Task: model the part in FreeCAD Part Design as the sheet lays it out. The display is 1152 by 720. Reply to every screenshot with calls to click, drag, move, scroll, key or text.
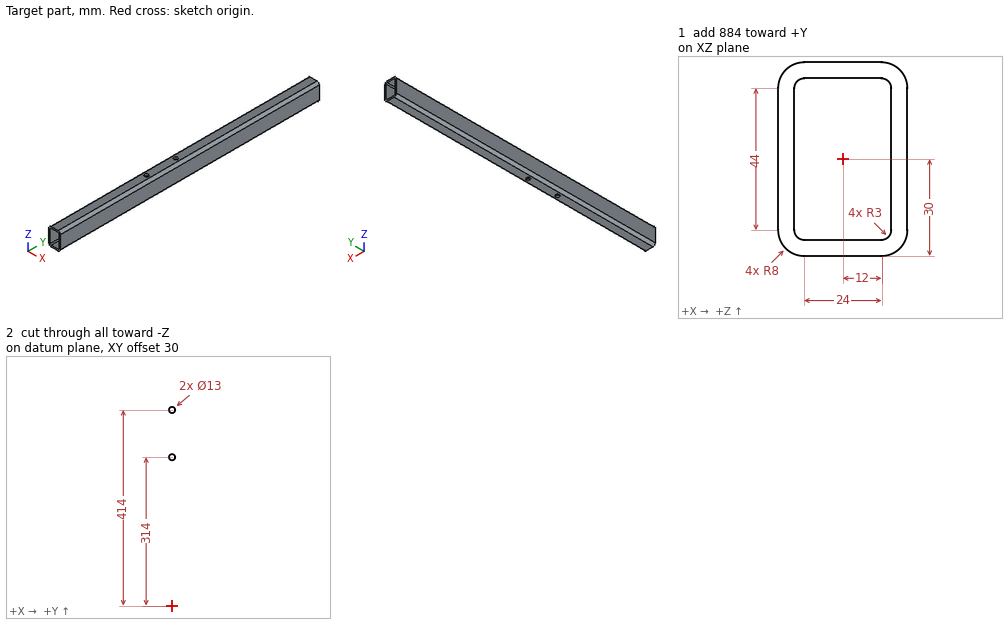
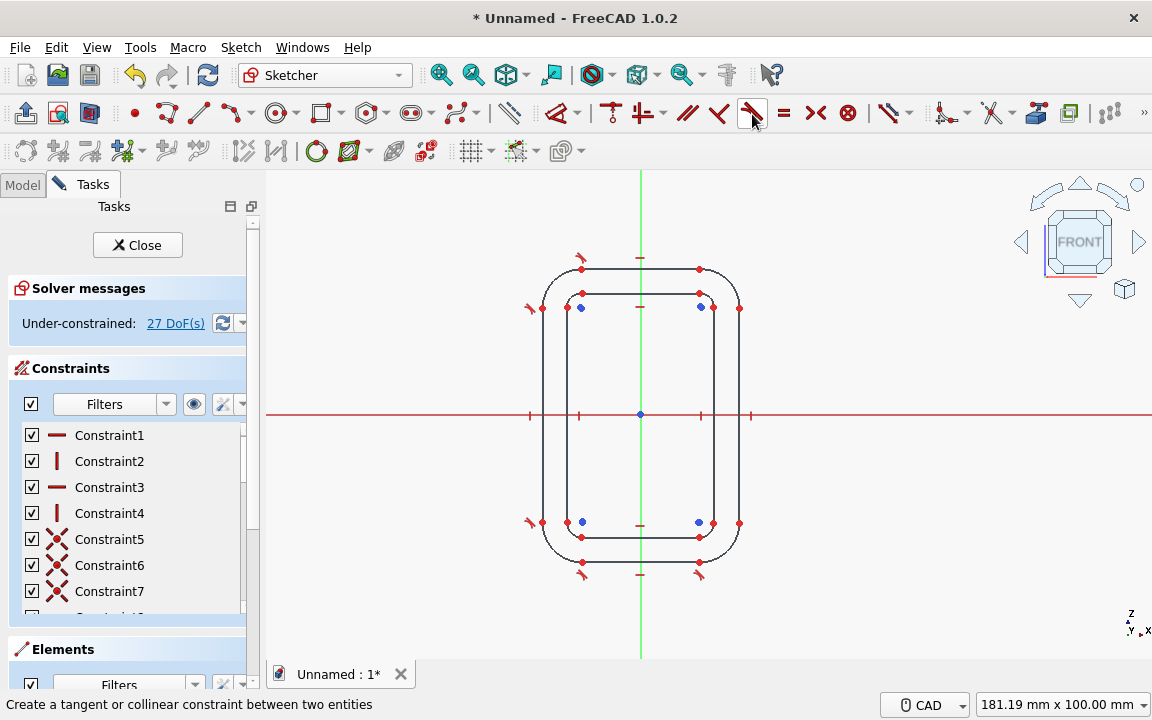
click(617, 269)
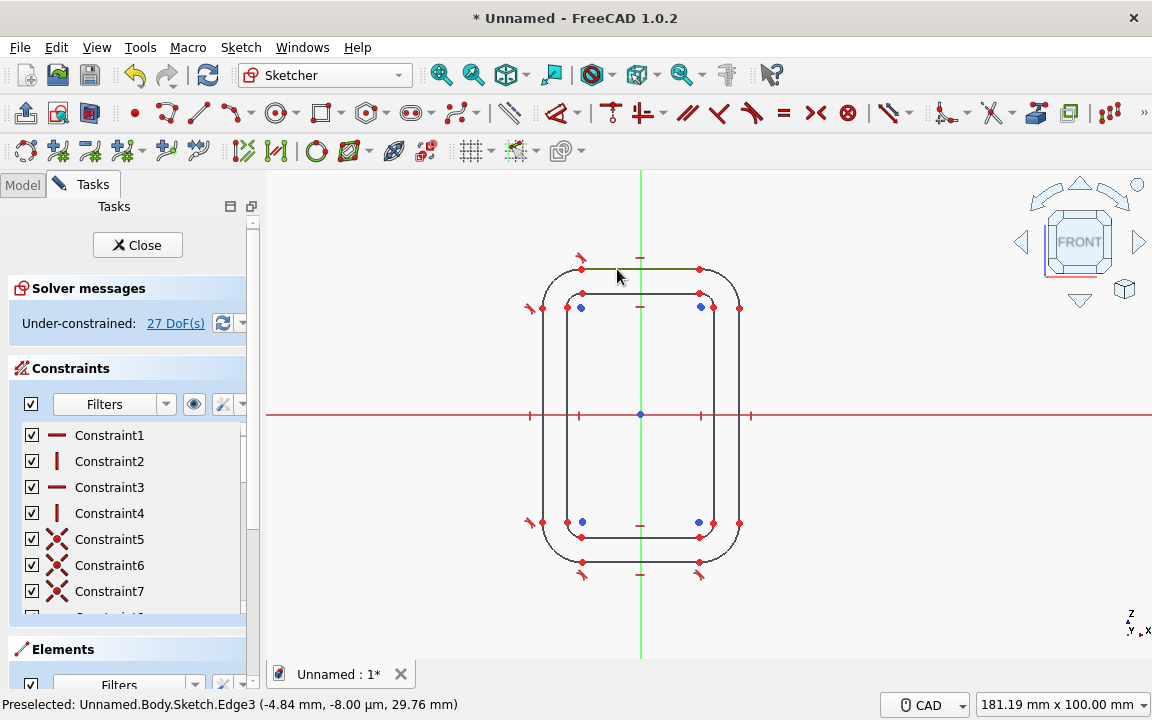
click(735, 290)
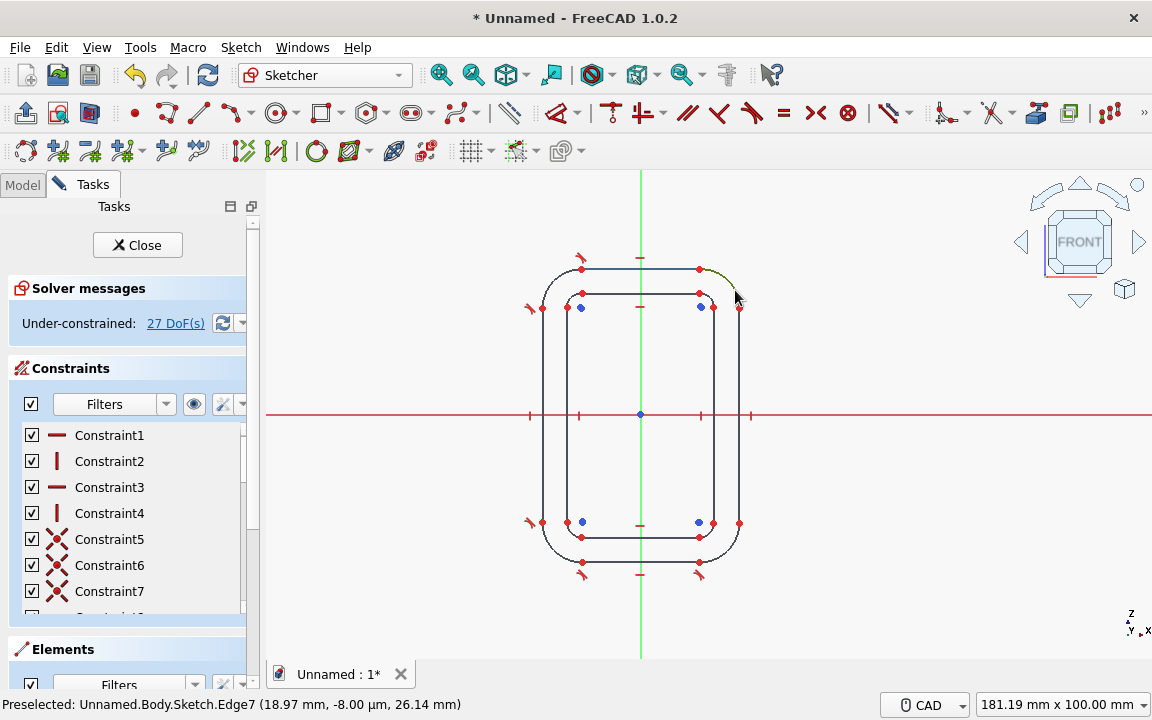
key(t)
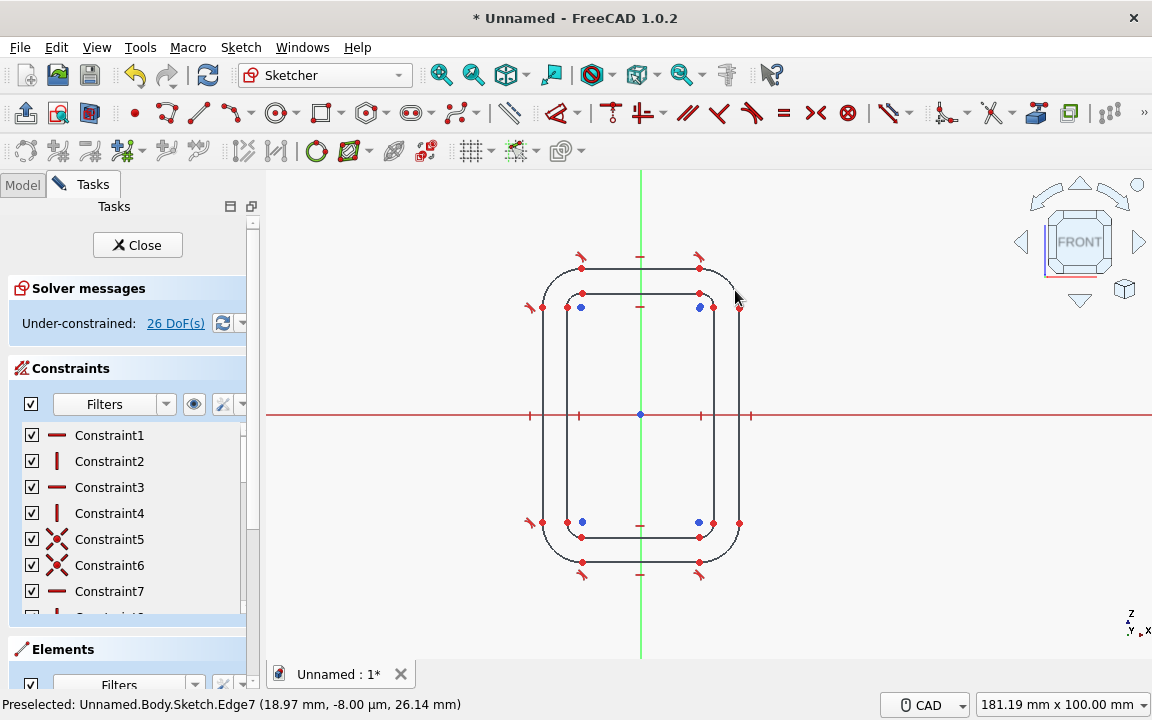
click(739, 373)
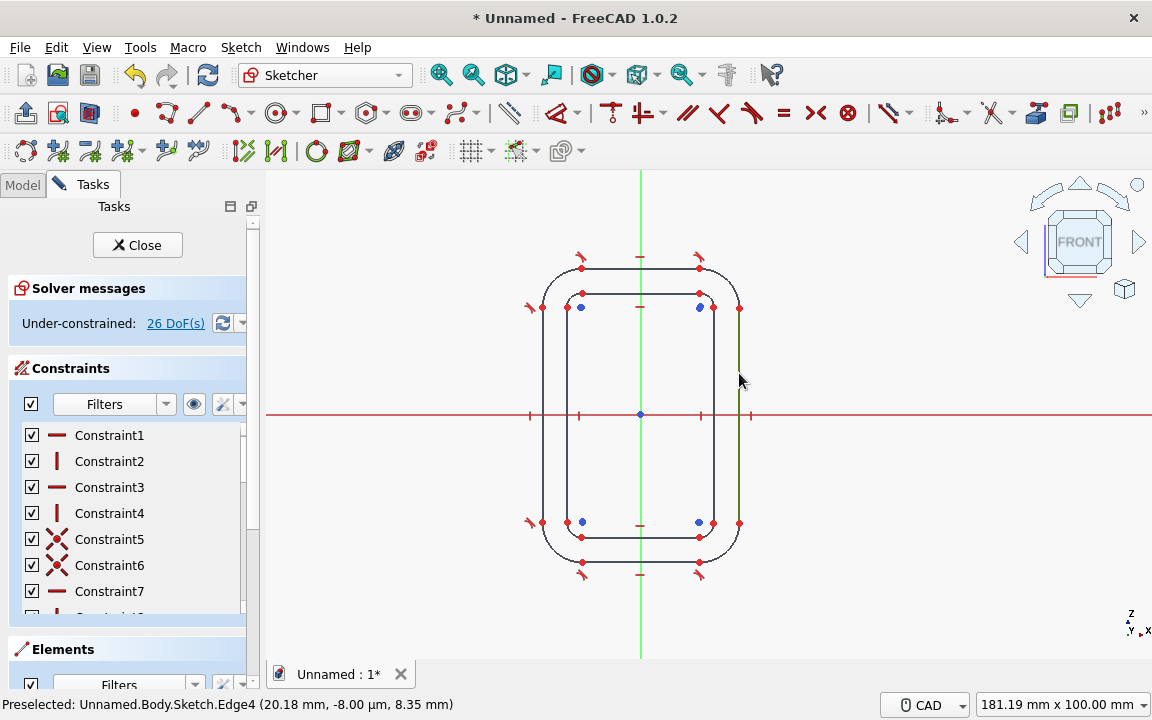
click(735, 290)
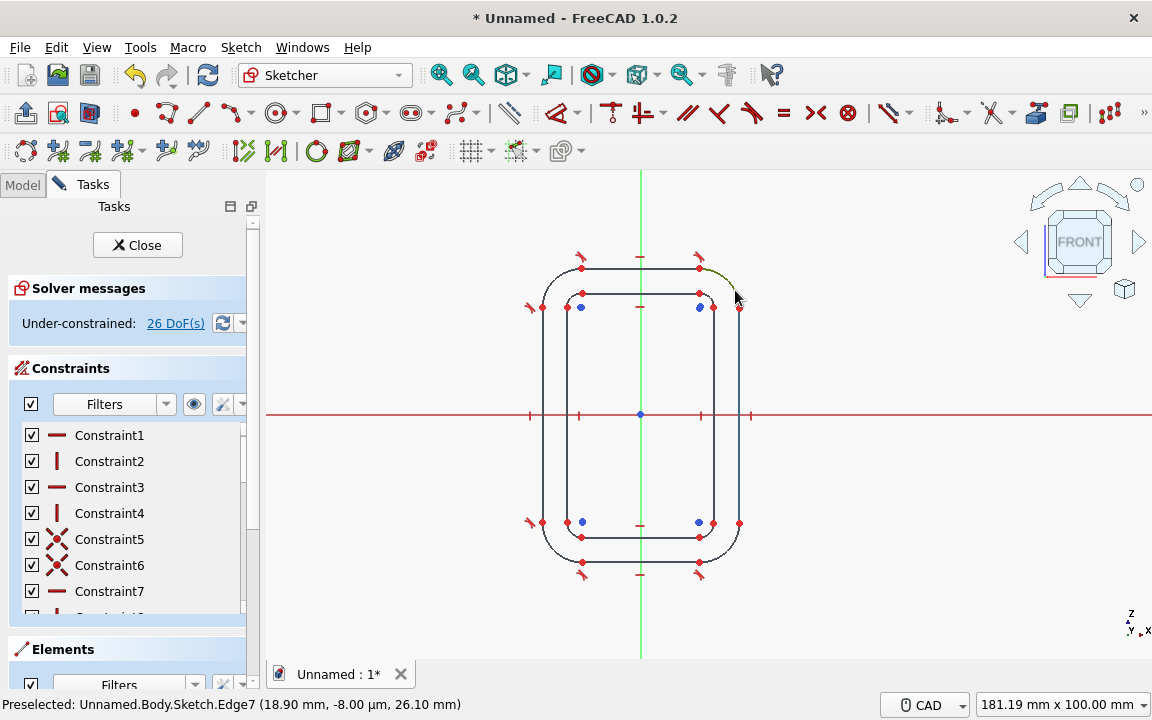
click(752, 114)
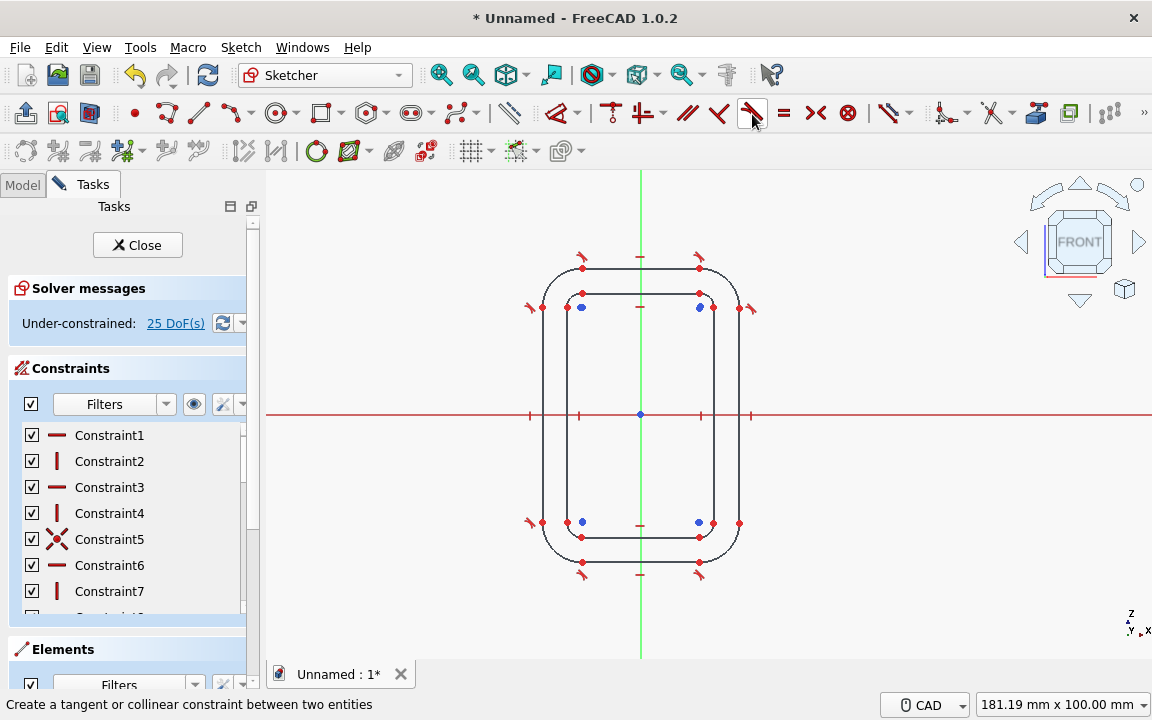
click(739, 373)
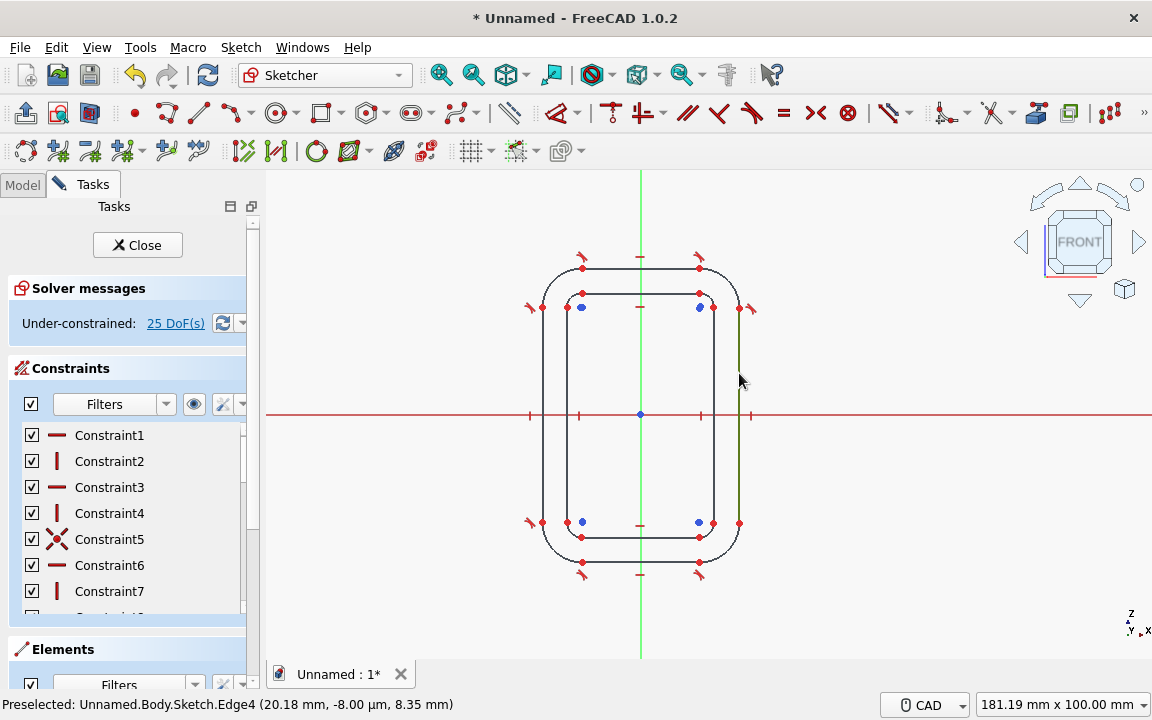
click(718, 558)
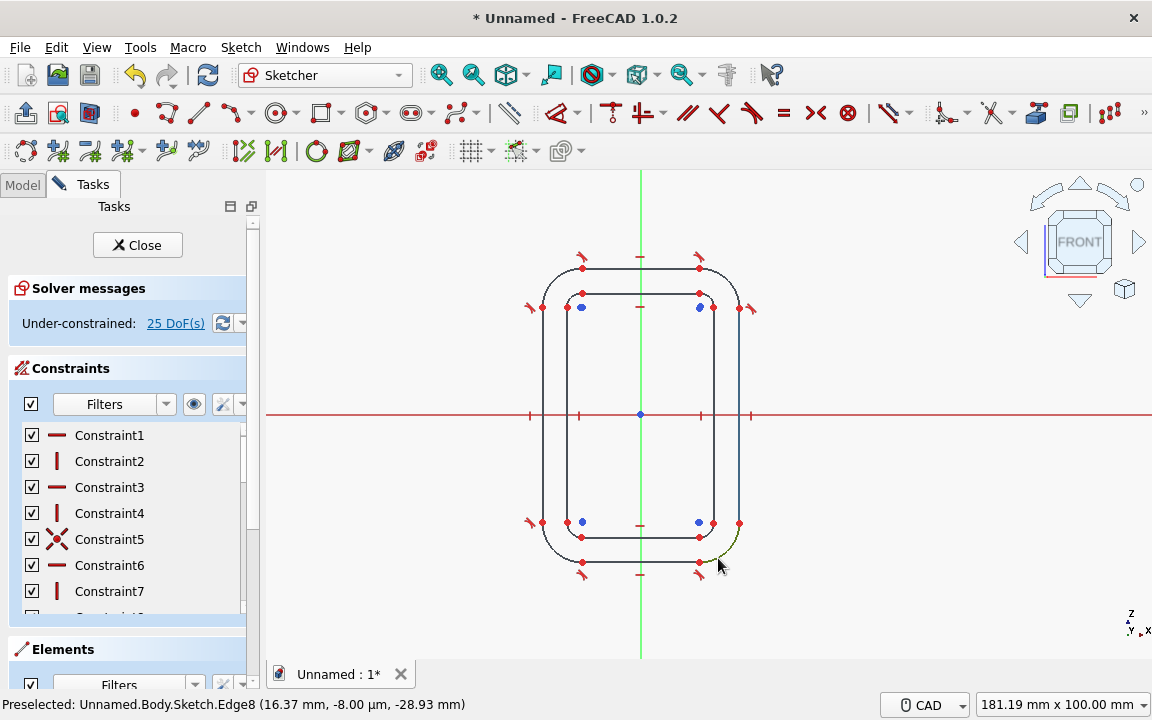
key(t)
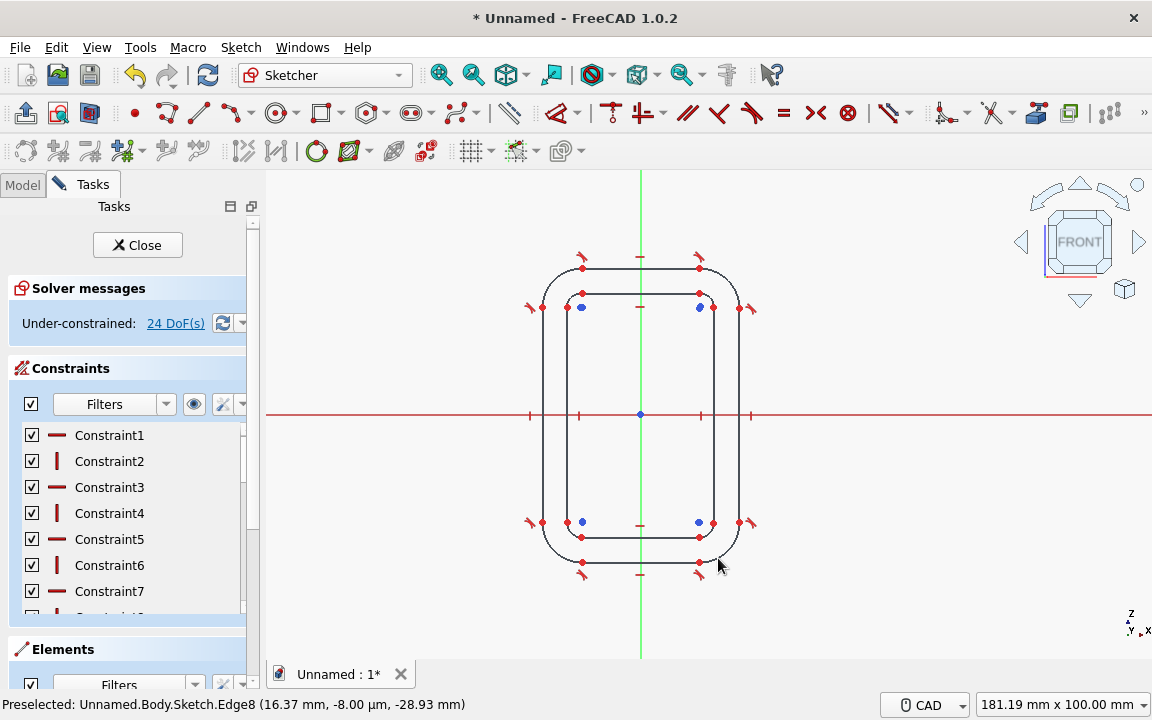
click(617, 538)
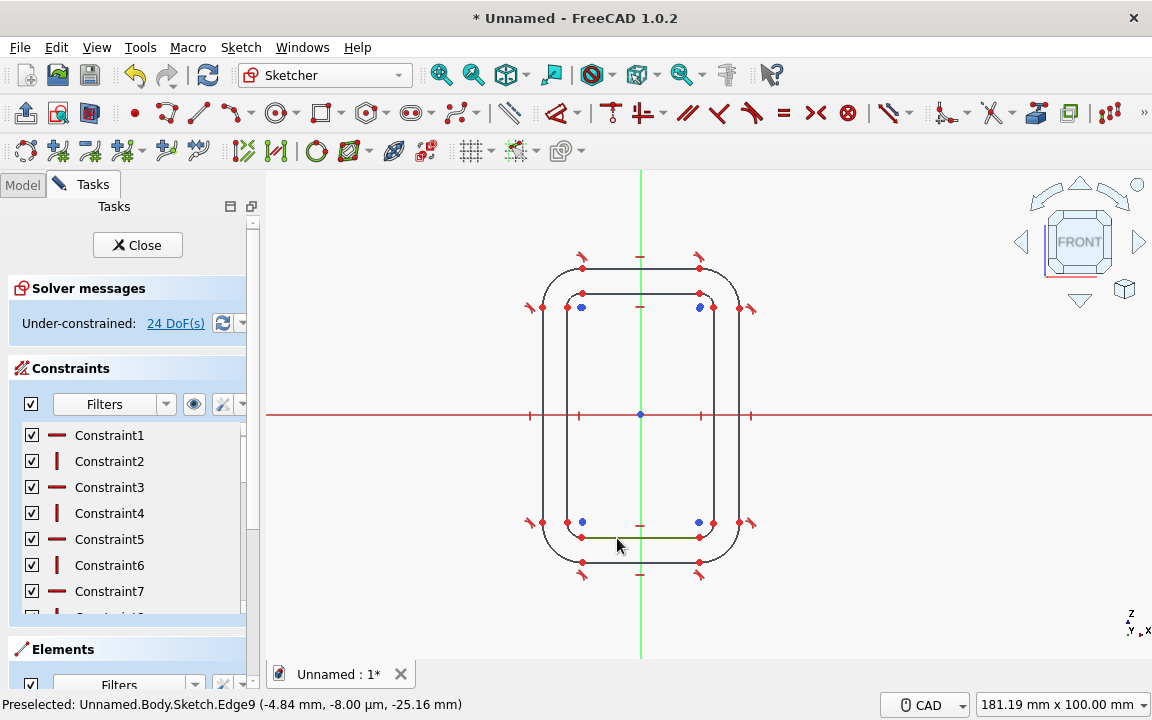
scroll(710, 533, up, 2)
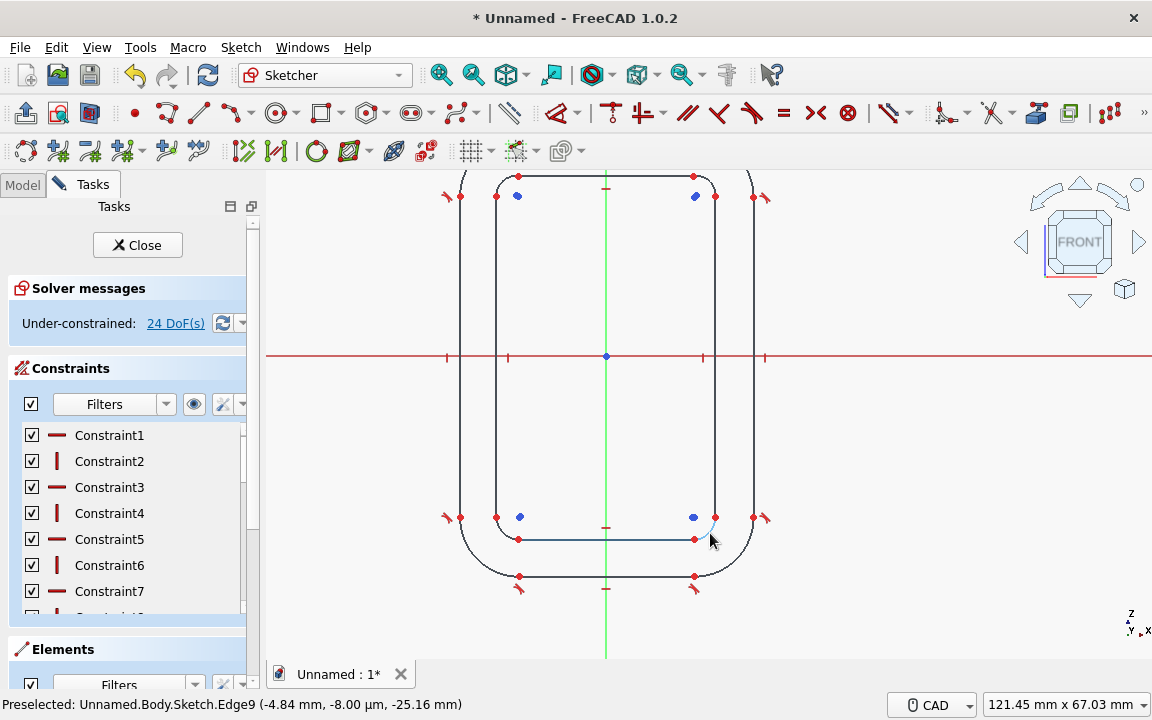
click(709, 533)